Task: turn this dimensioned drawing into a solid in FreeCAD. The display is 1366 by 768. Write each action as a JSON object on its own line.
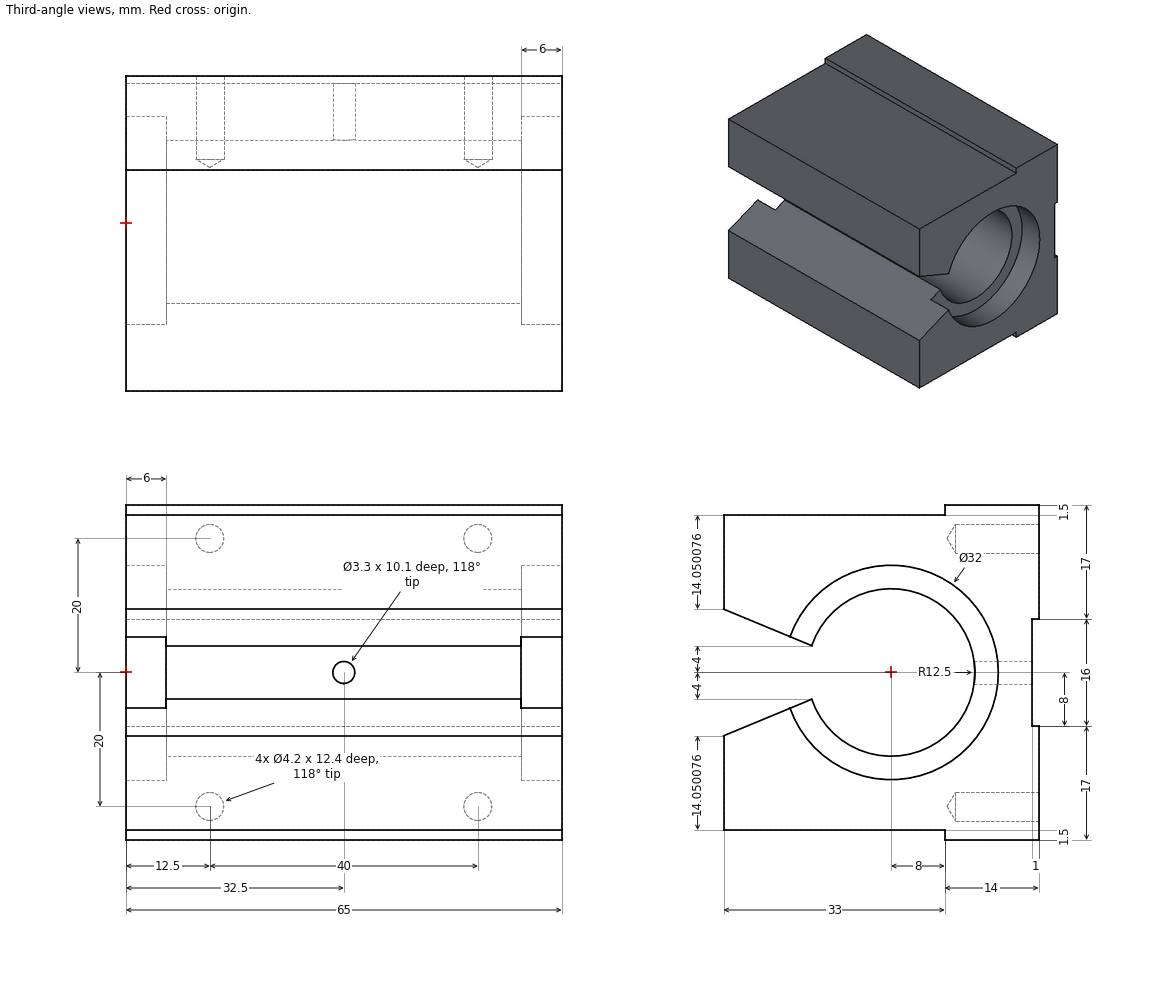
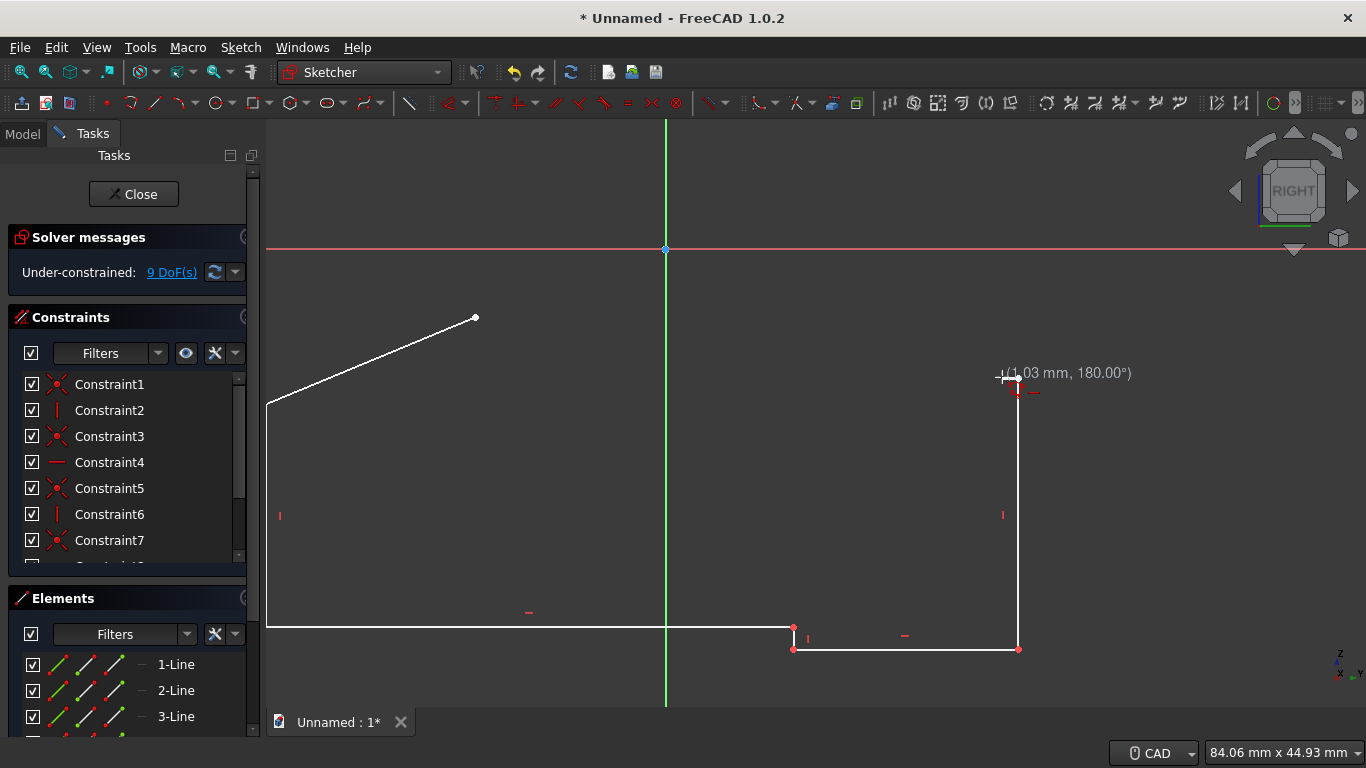
{"action": "left_click", "coordinate": [1002, 377]}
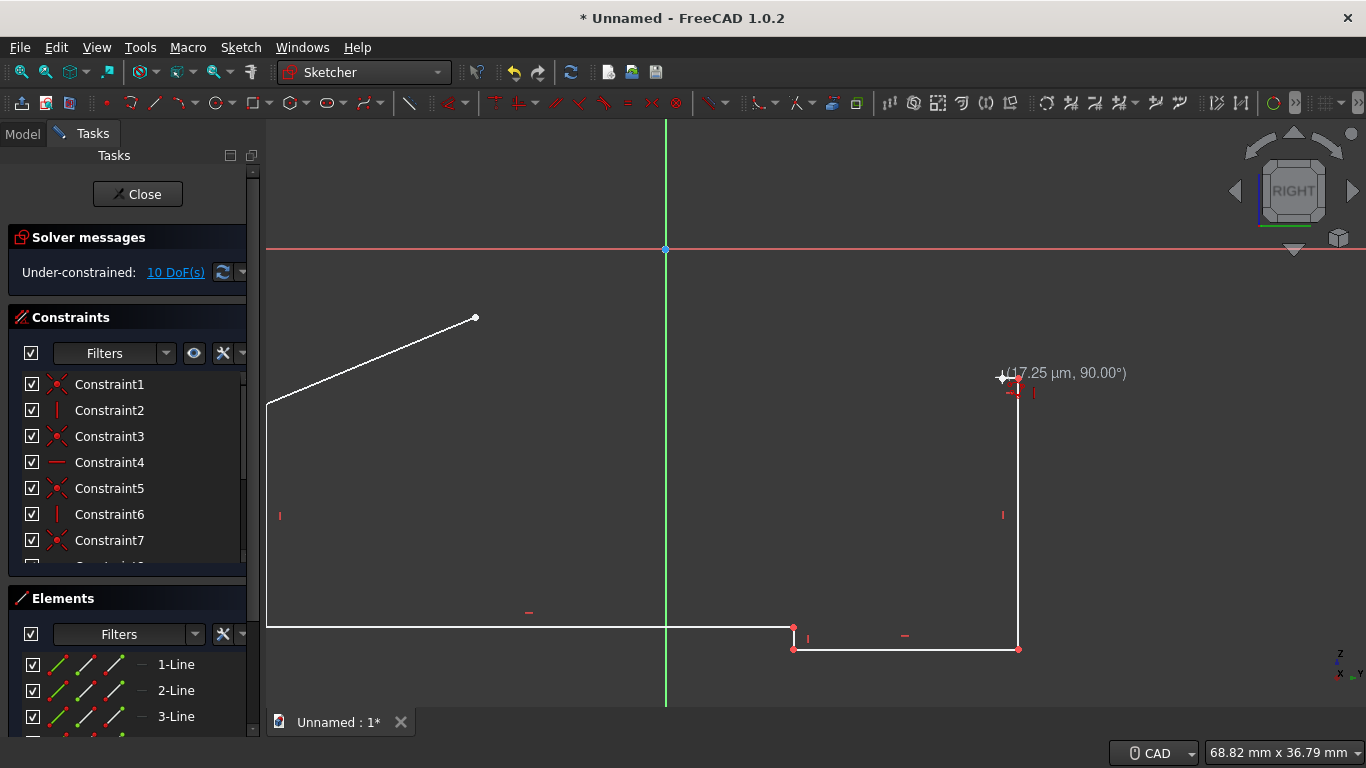
{"action": "scroll", "coordinate": [834, 547], "scroll_direction": "down", "scroll_amount": 4}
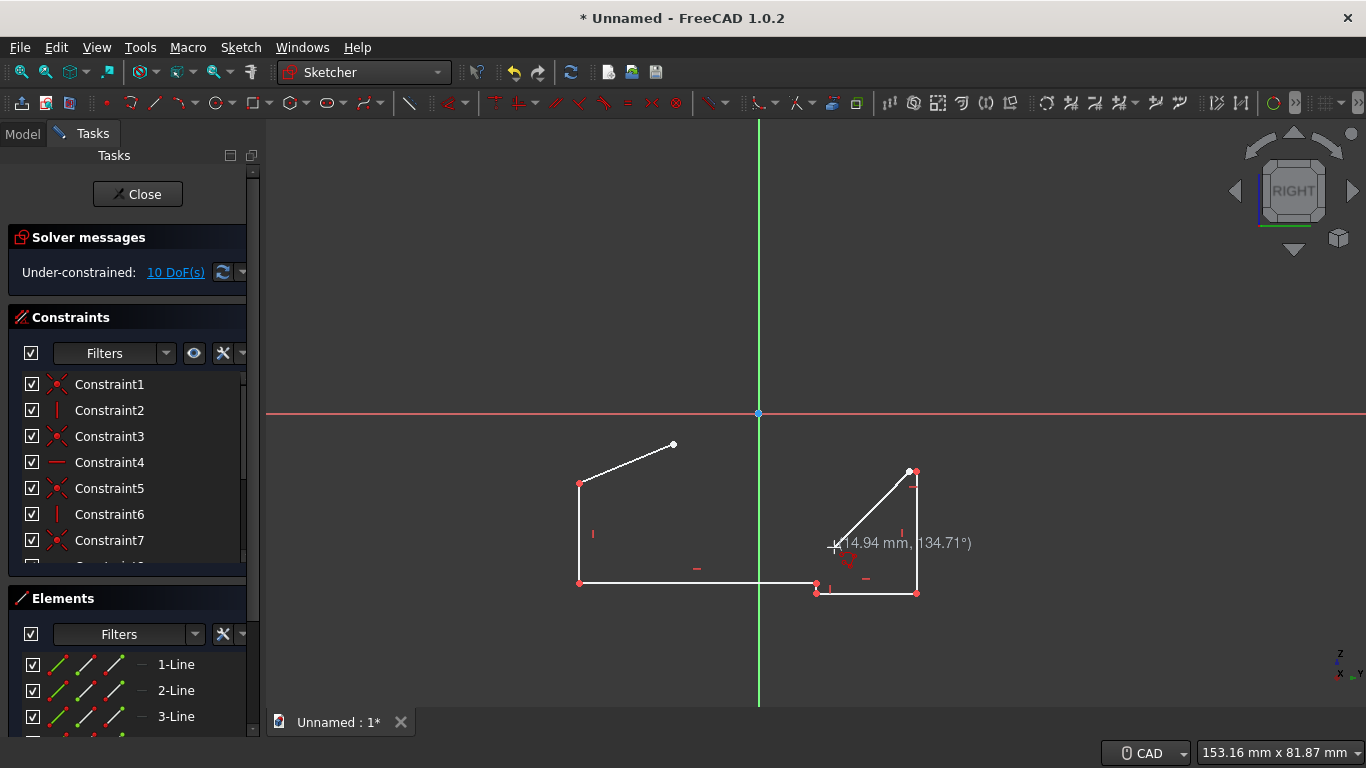
{"action": "left_click", "coordinate": [910, 356]}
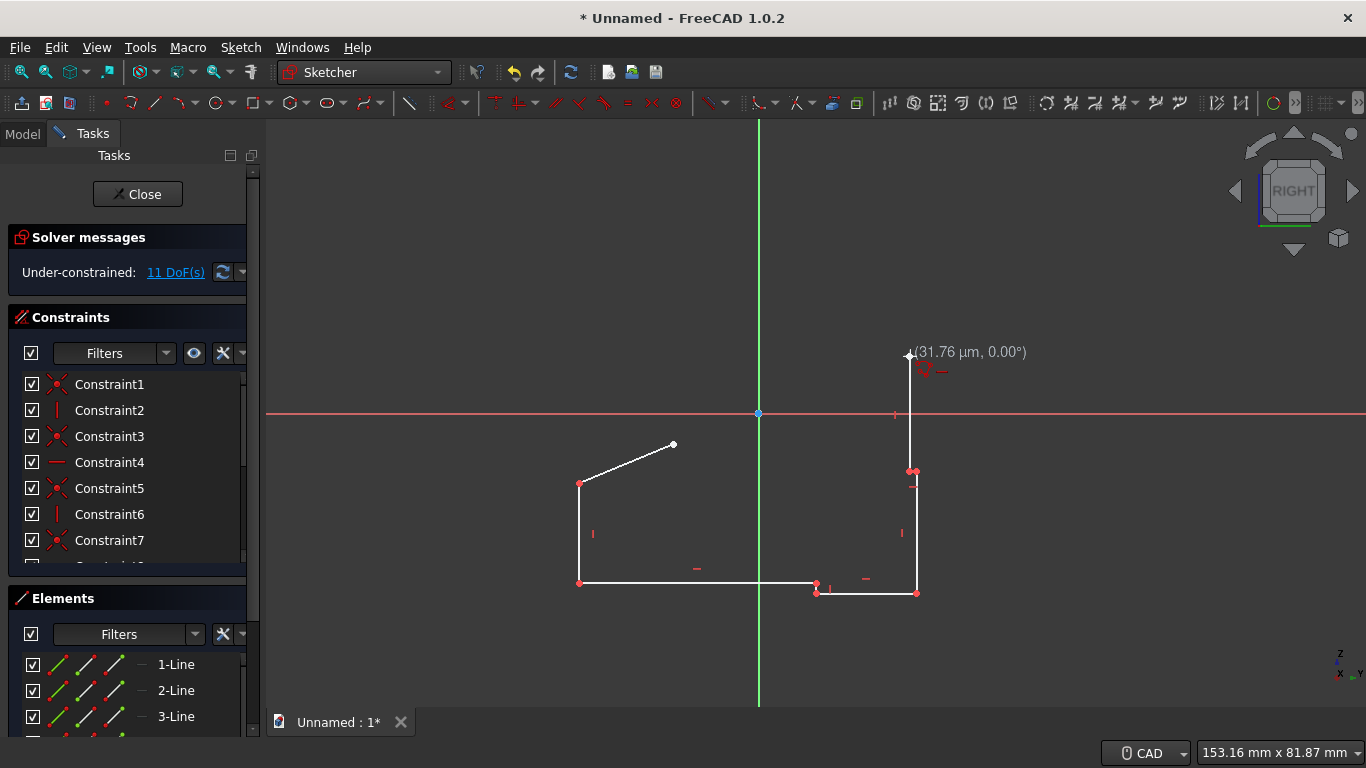
{"action": "scroll", "coordinate": [917, 356], "scroll_direction": "up", "scroll_amount": 4}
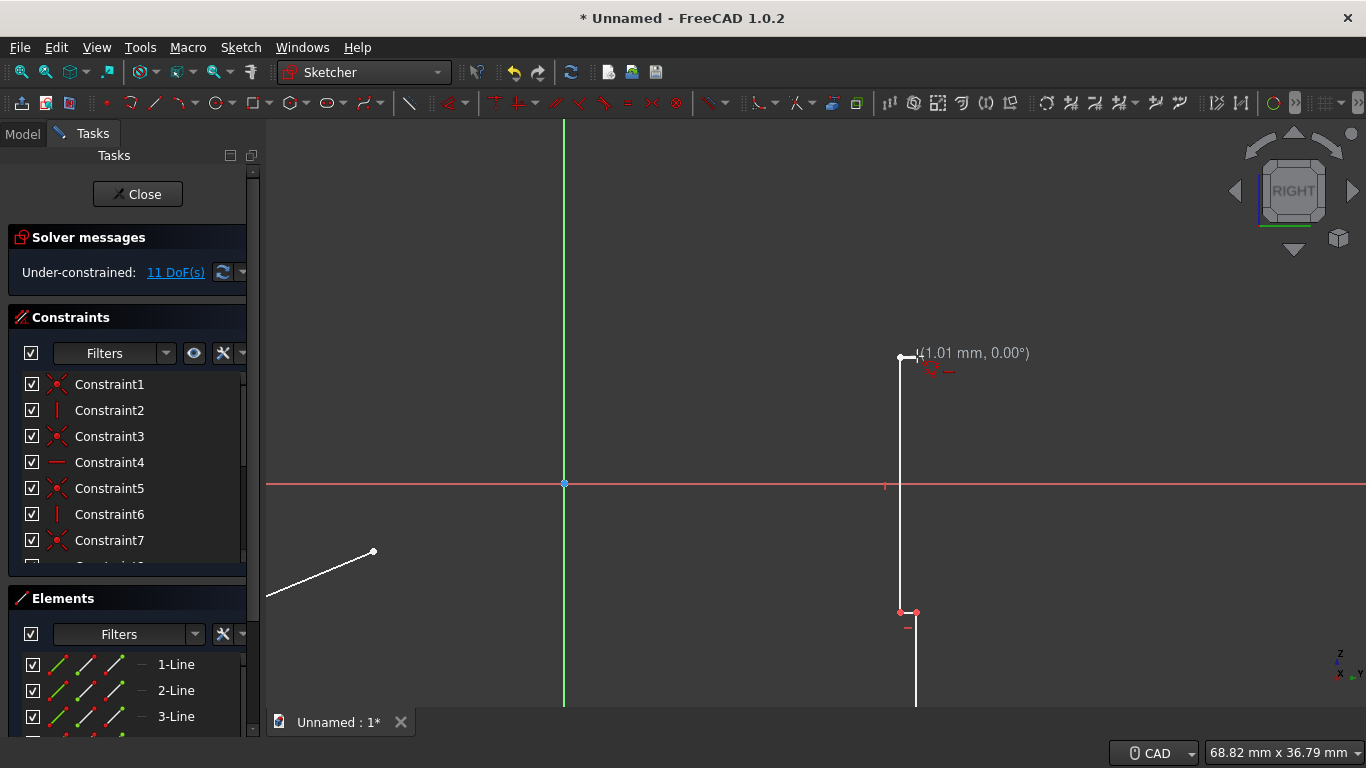
{"action": "left_click", "coordinate": [916, 356]}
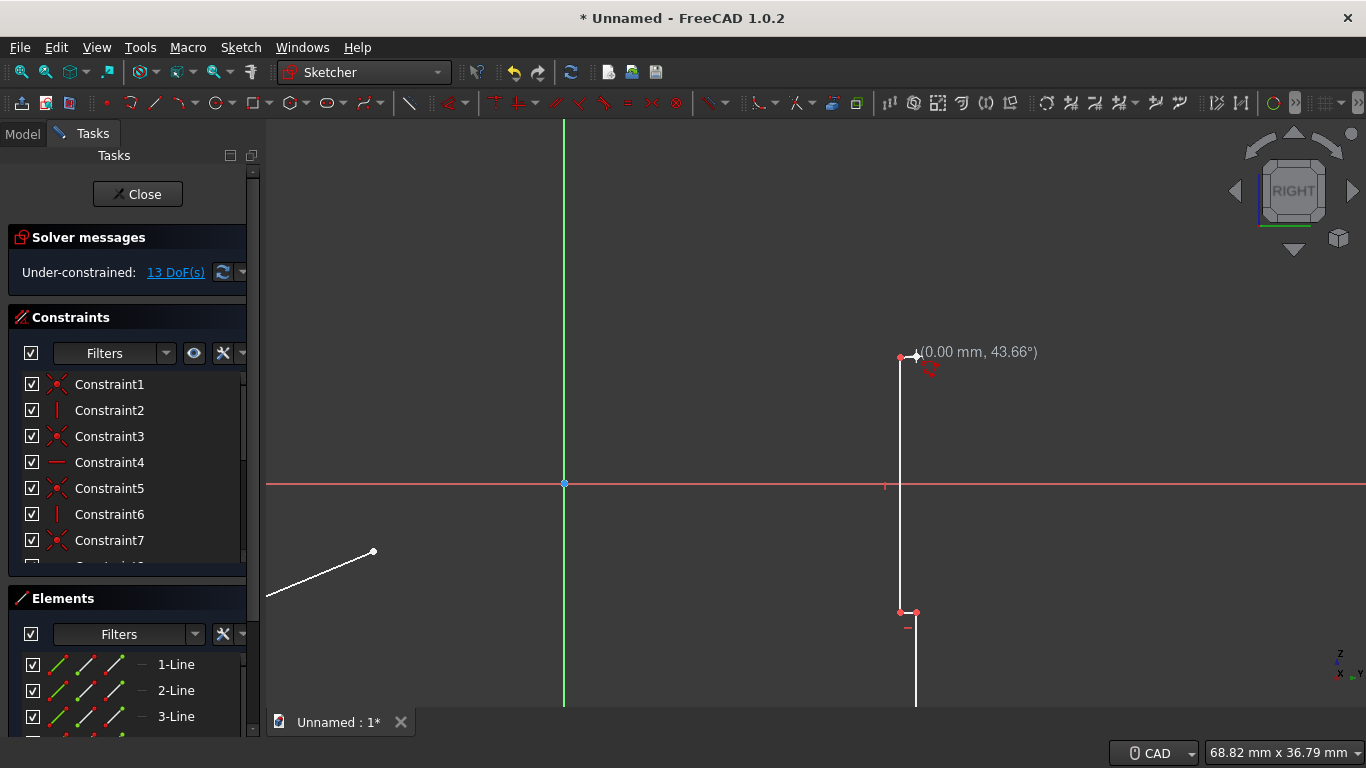
{"action": "scroll", "coordinate": [917, 355], "scroll_direction": "down", "scroll_amount": 4}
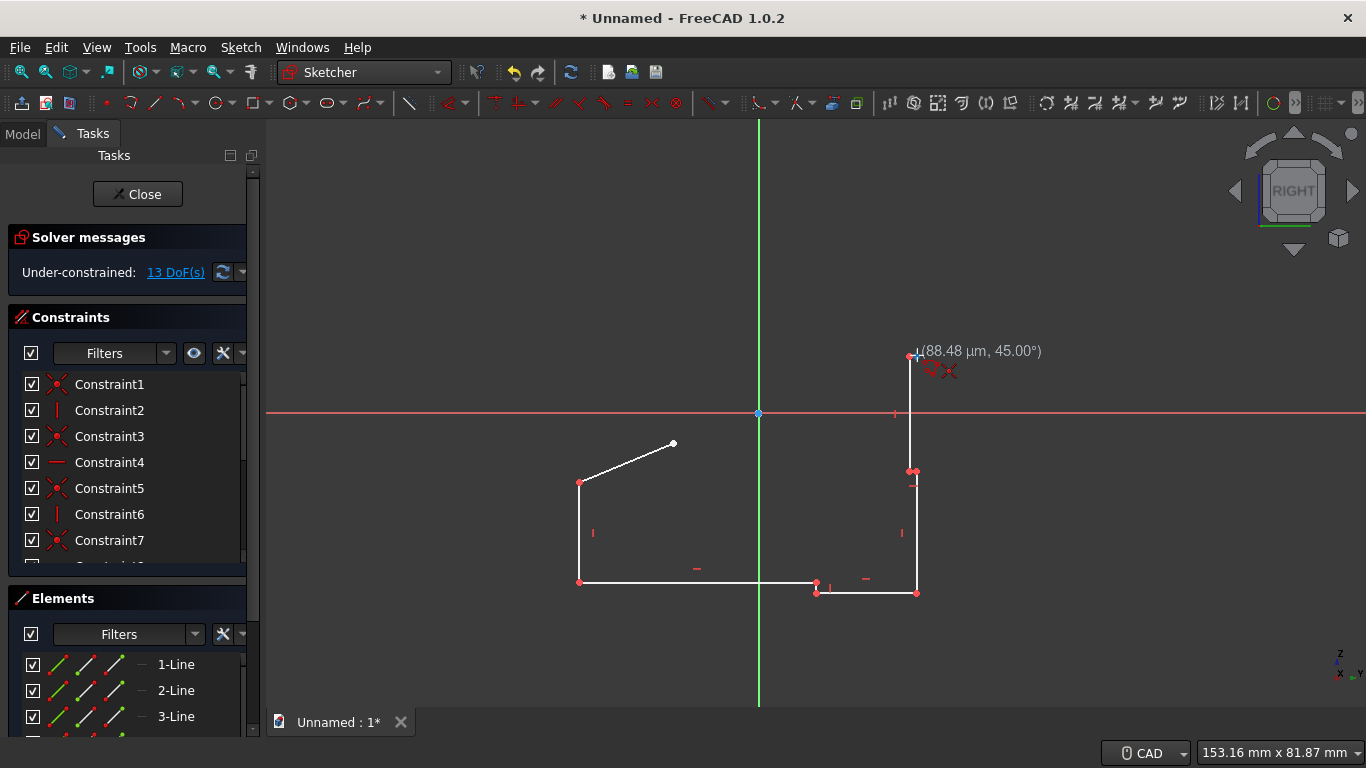
{"action": "left_click", "coordinate": [917, 234]}
{"action": "left_click", "coordinate": [816, 234]}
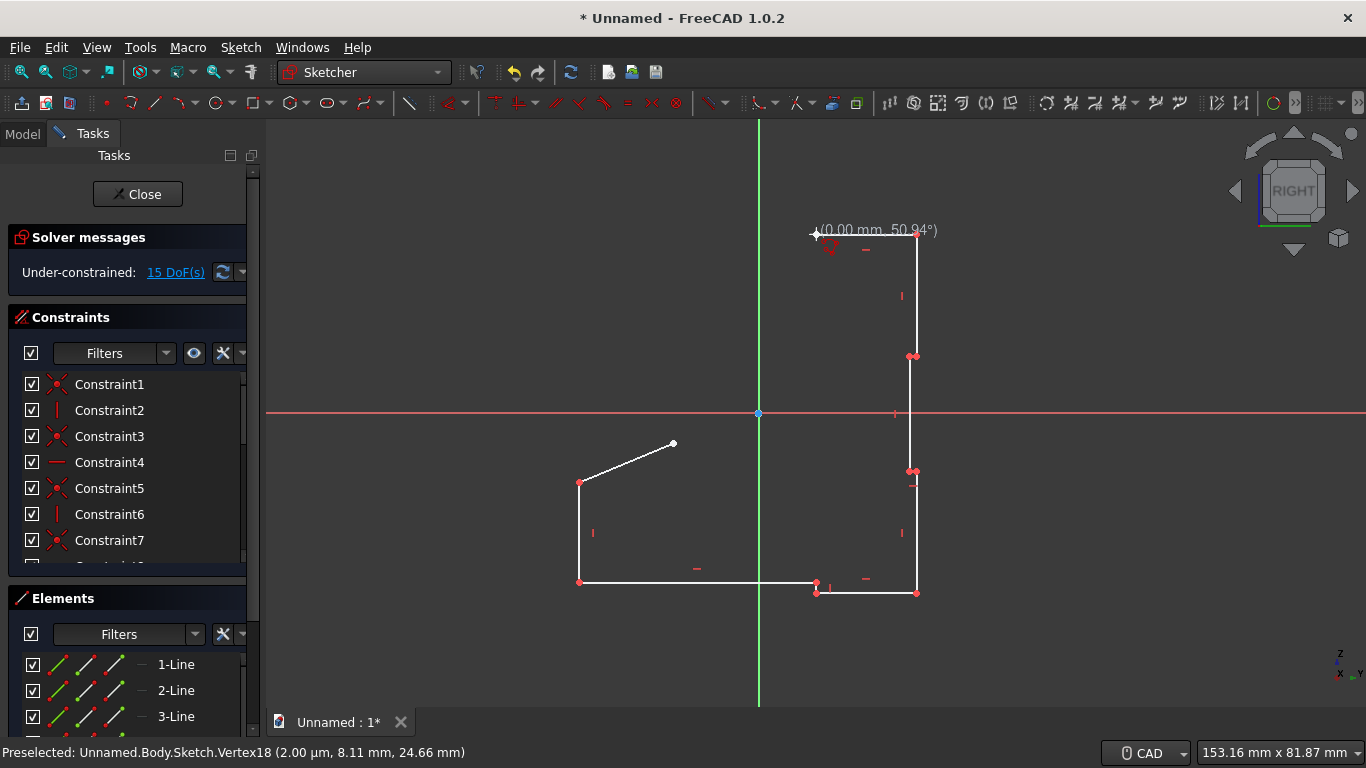
{"action": "scroll", "coordinate": [816, 244], "scroll_direction": "up", "scroll_amount": 2}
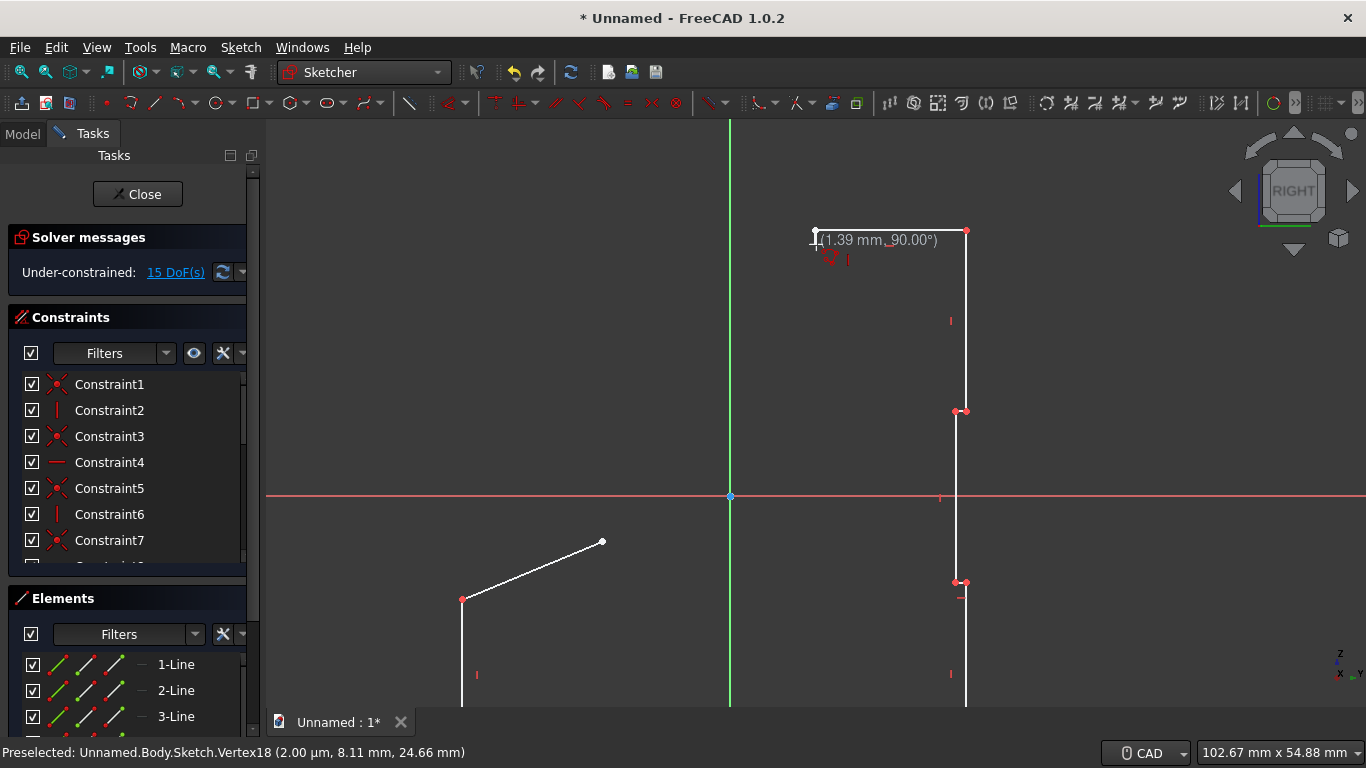
{"action": "left_click", "coordinate": [816, 244]}
{"action": "left_click", "coordinate": [462, 244]}
{"action": "left_click", "coordinate": [462, 395]}
{"action": "left_click", "coordinate": [603, 453]}
{"action": "right_click", "coordinate": [603, 453]}